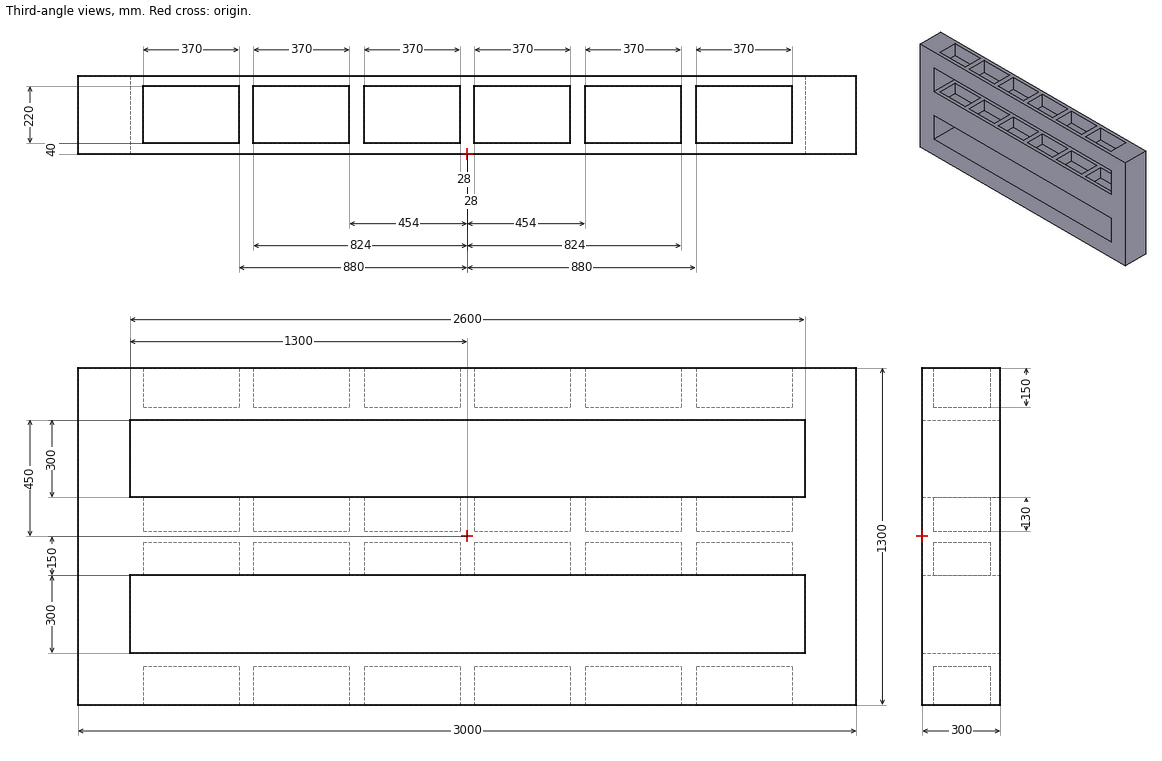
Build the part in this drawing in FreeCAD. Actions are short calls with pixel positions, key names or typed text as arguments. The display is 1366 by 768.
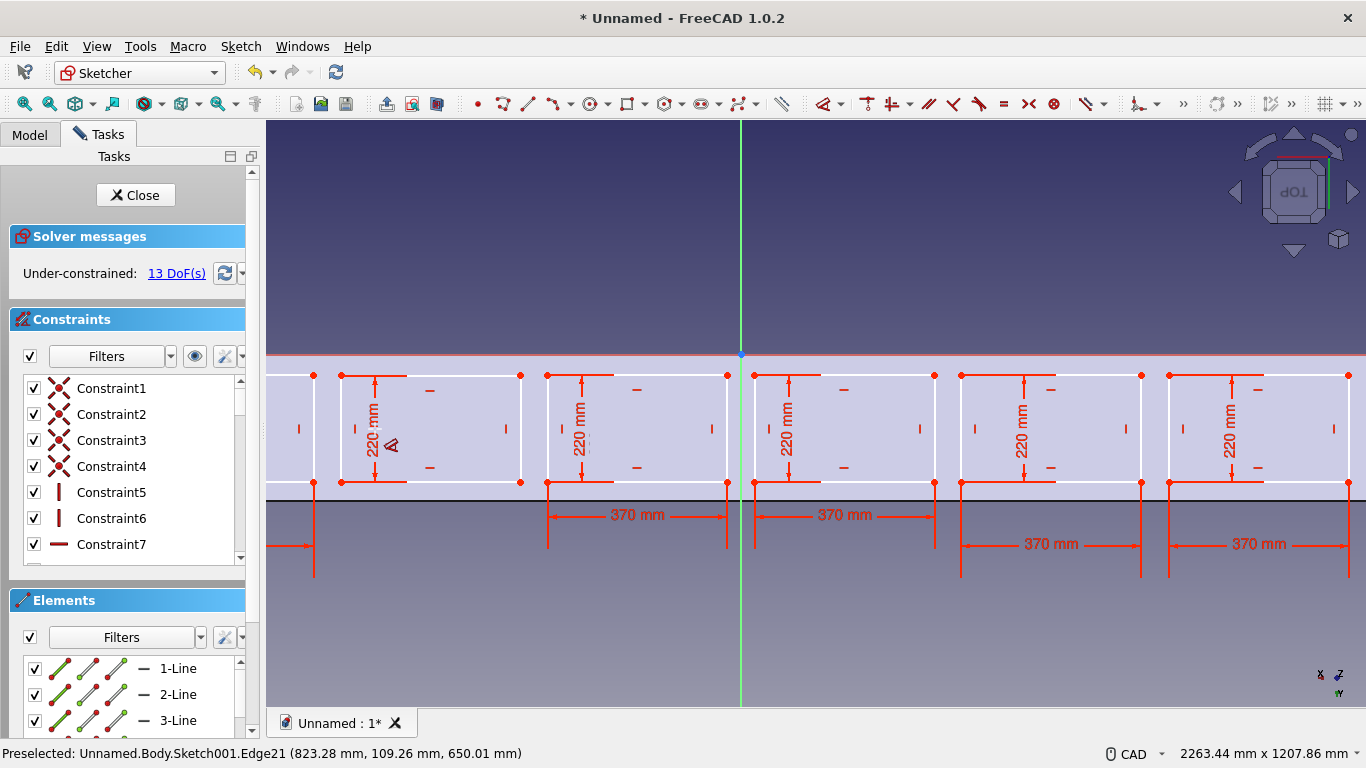
click(395, 482)
click(431, 516)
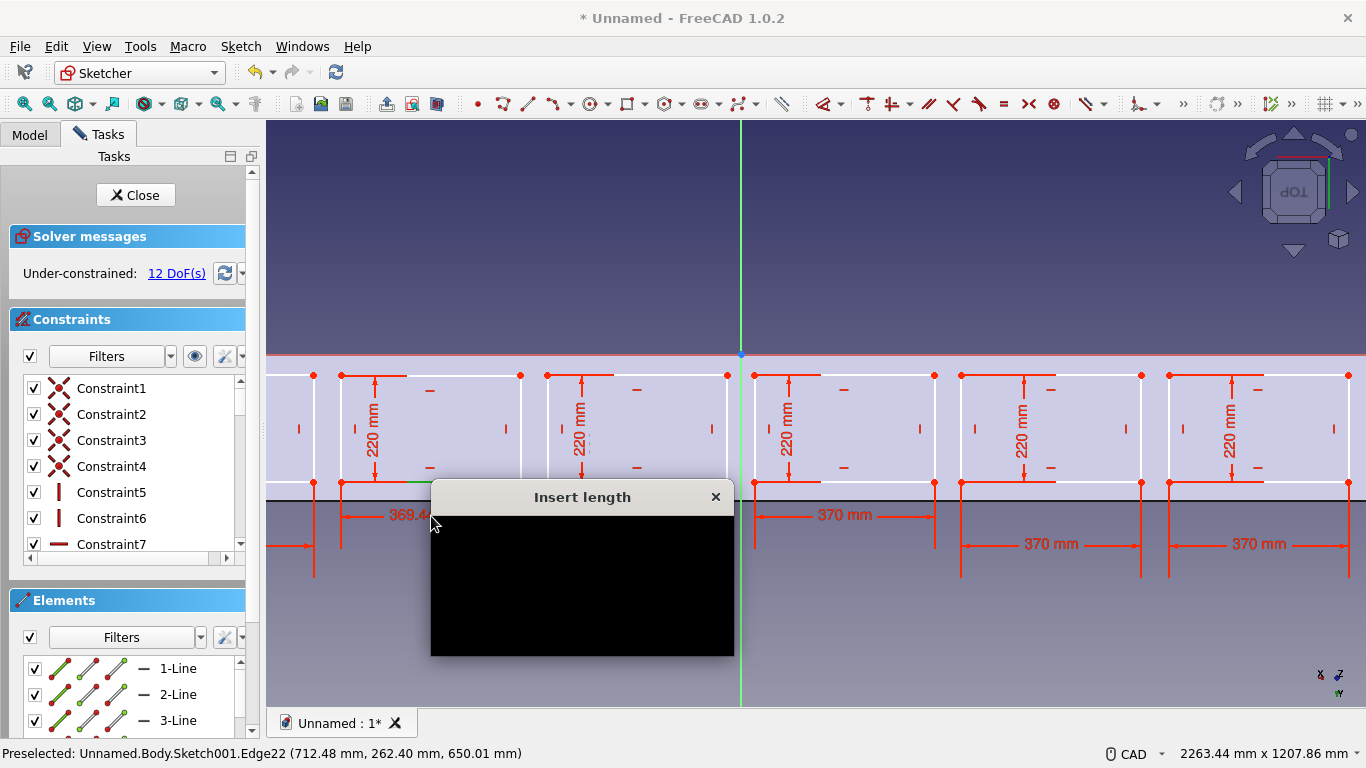
text(370)
key(Return)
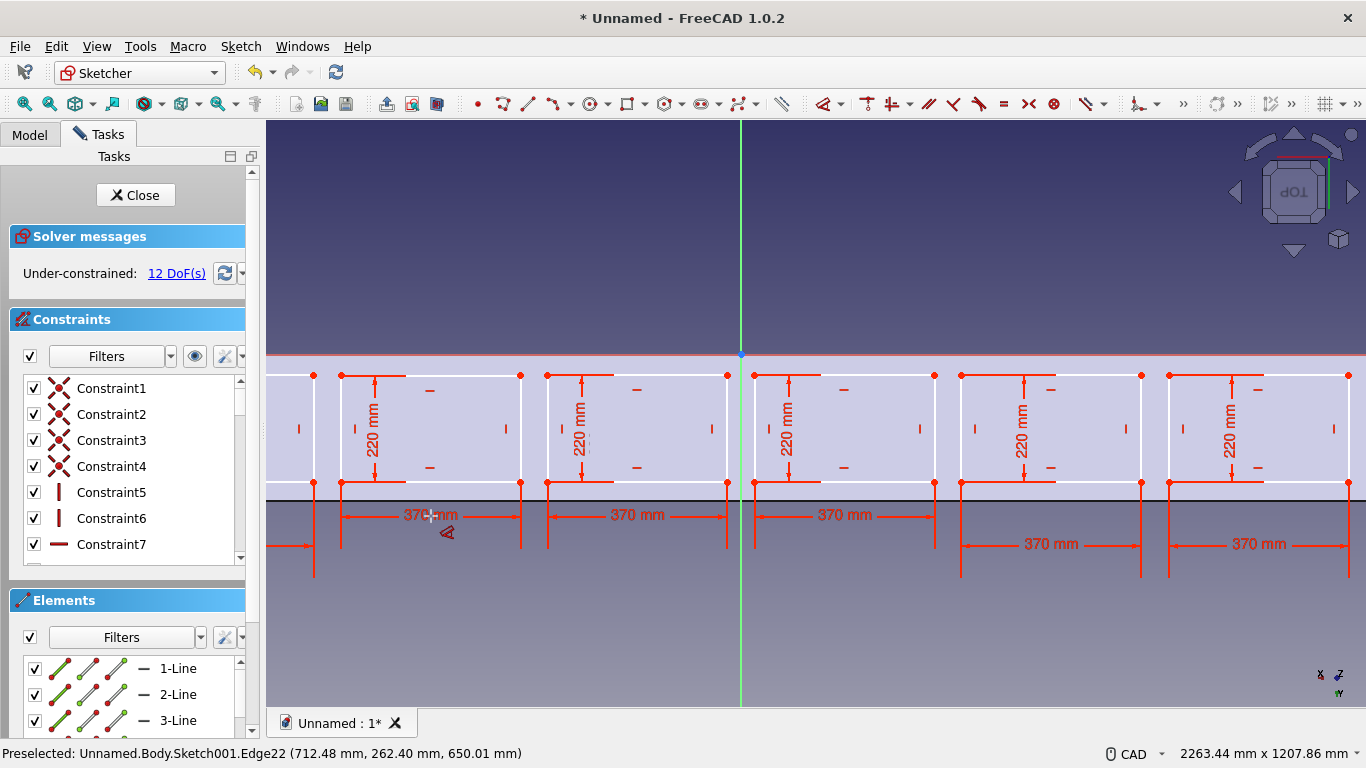
scroll(1169, 375, up, 4)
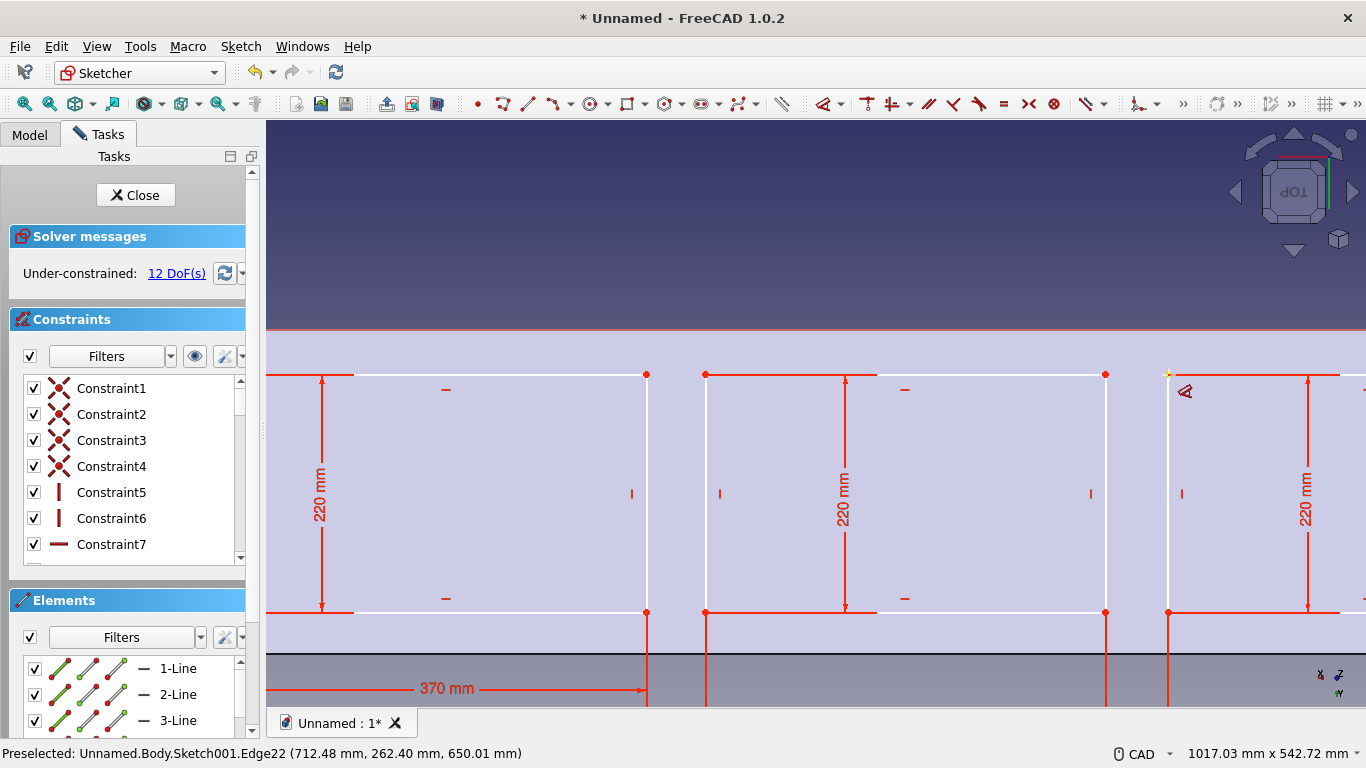
click(1168, 375)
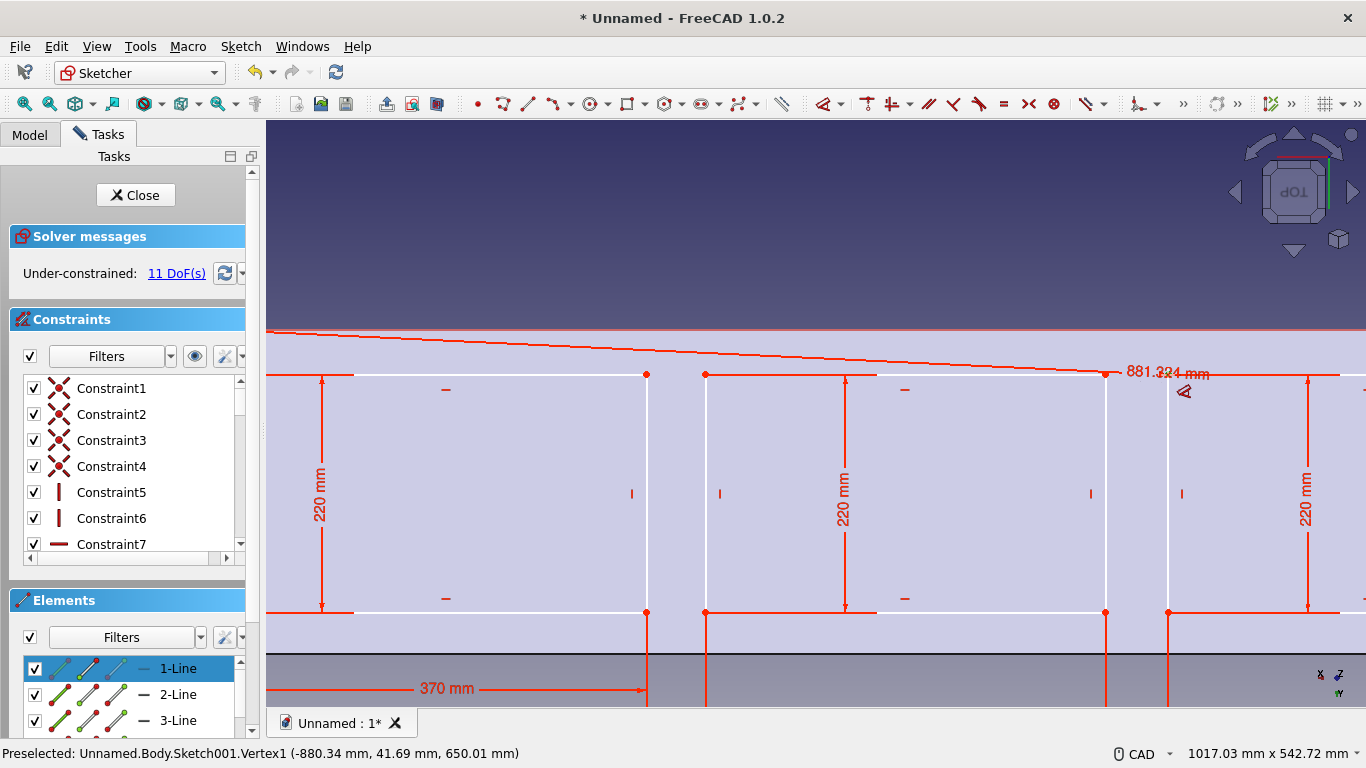
key(Escape)
key(Escape)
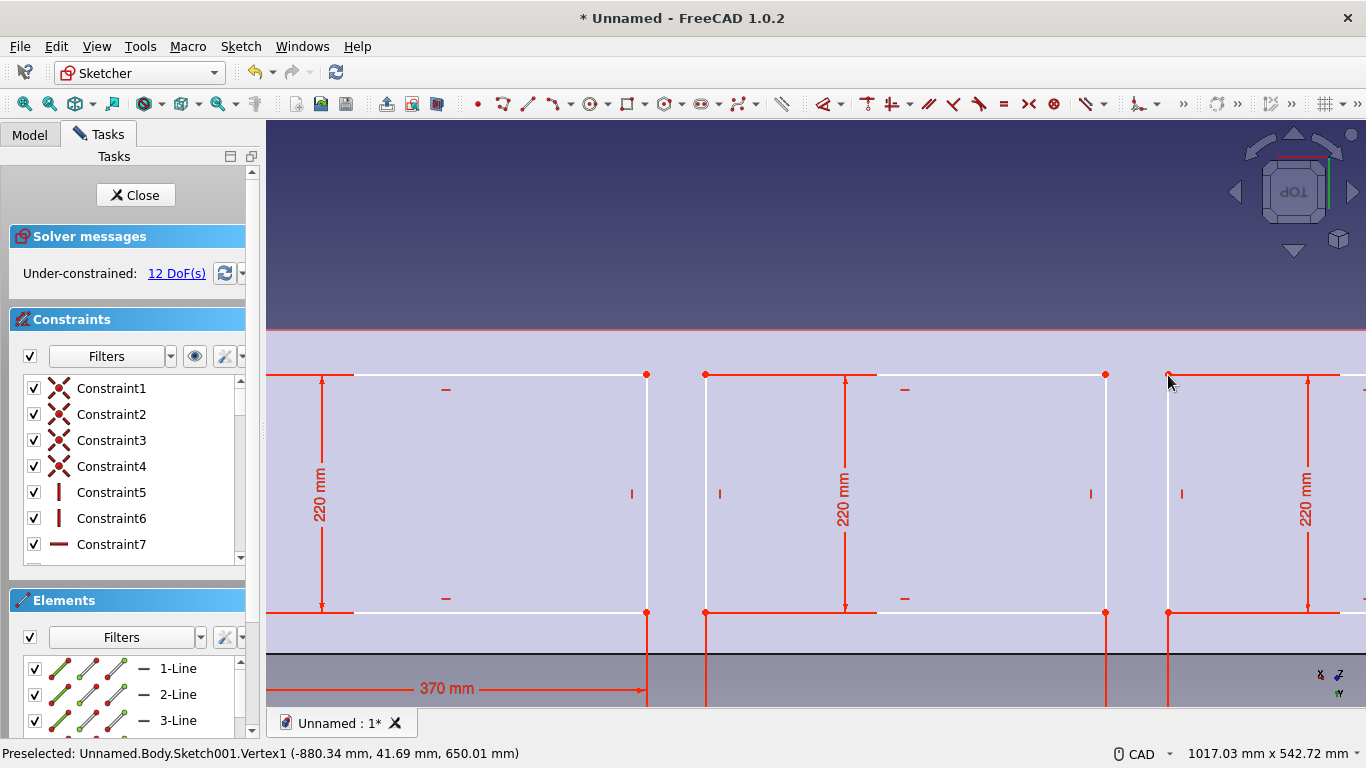
click(1168, 375)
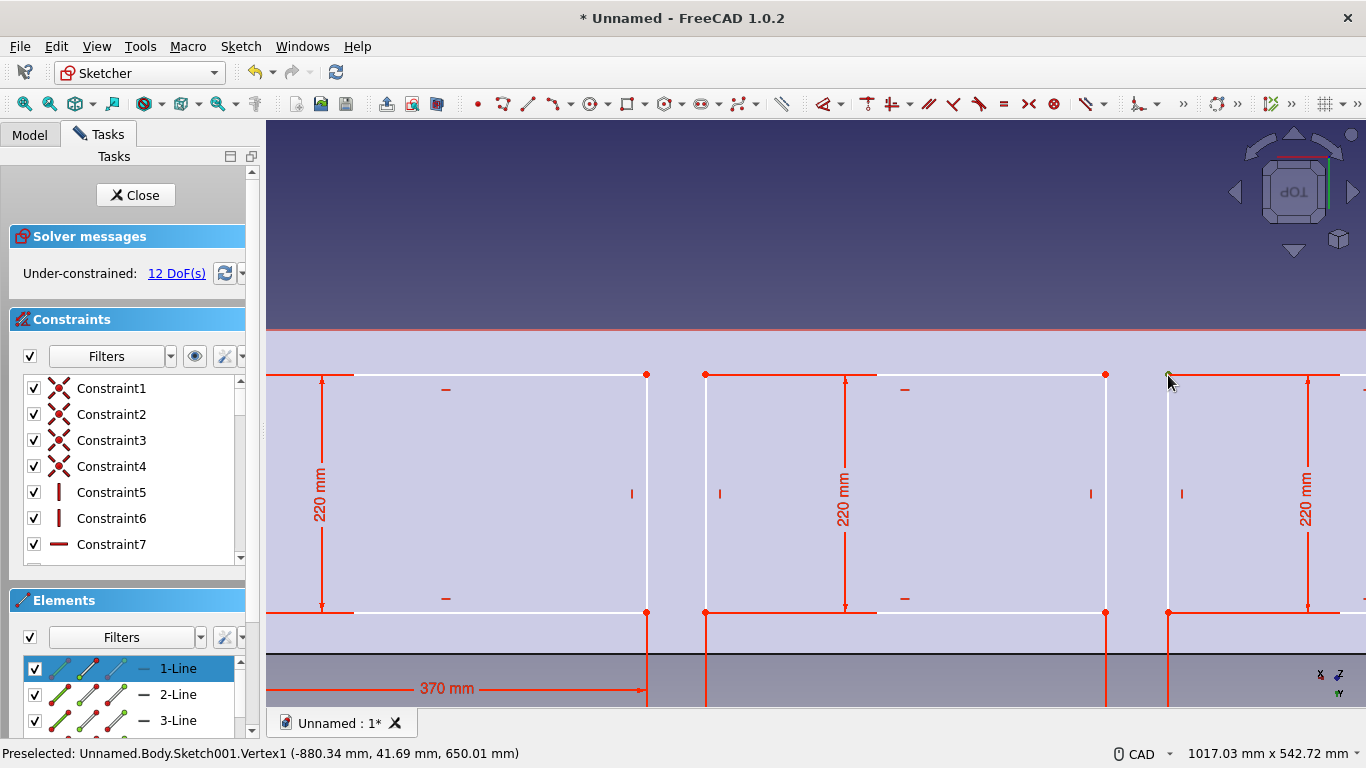
click(840, 104)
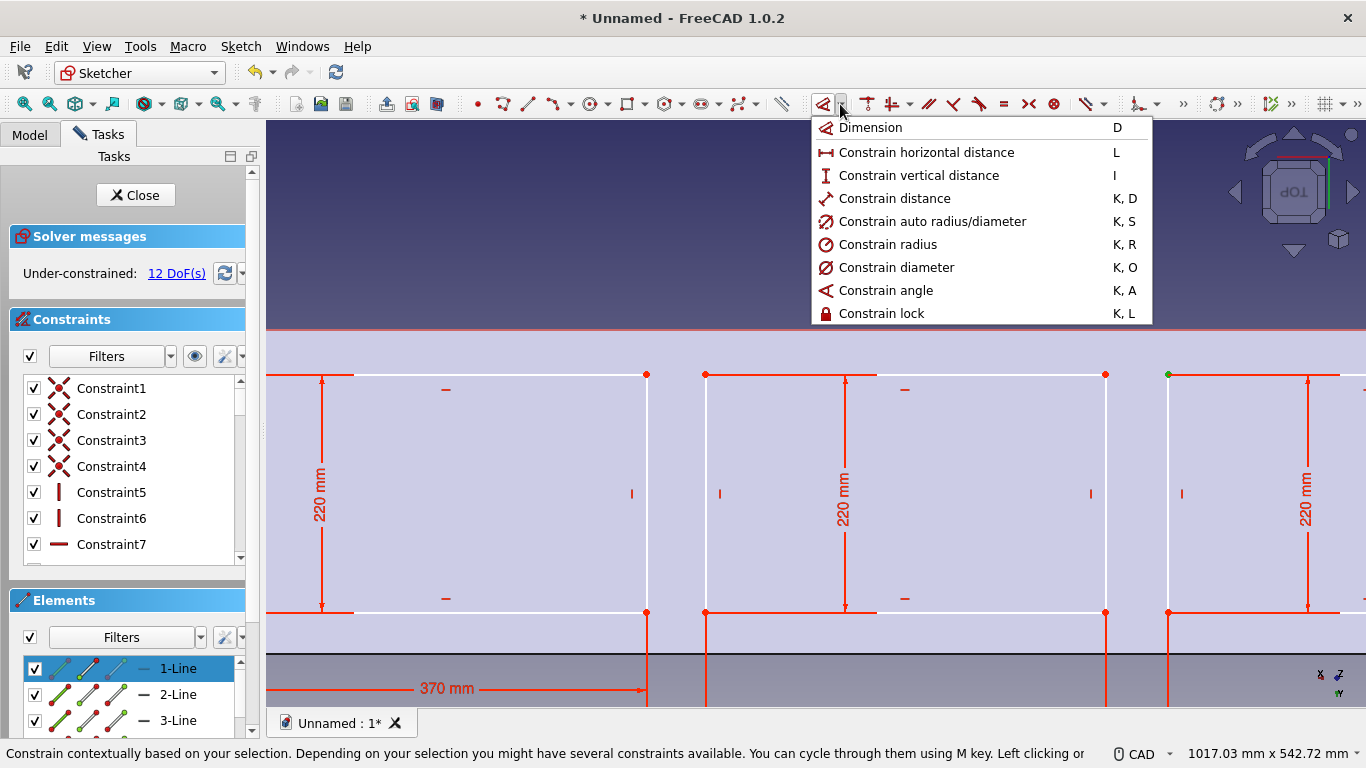
click(982, 176)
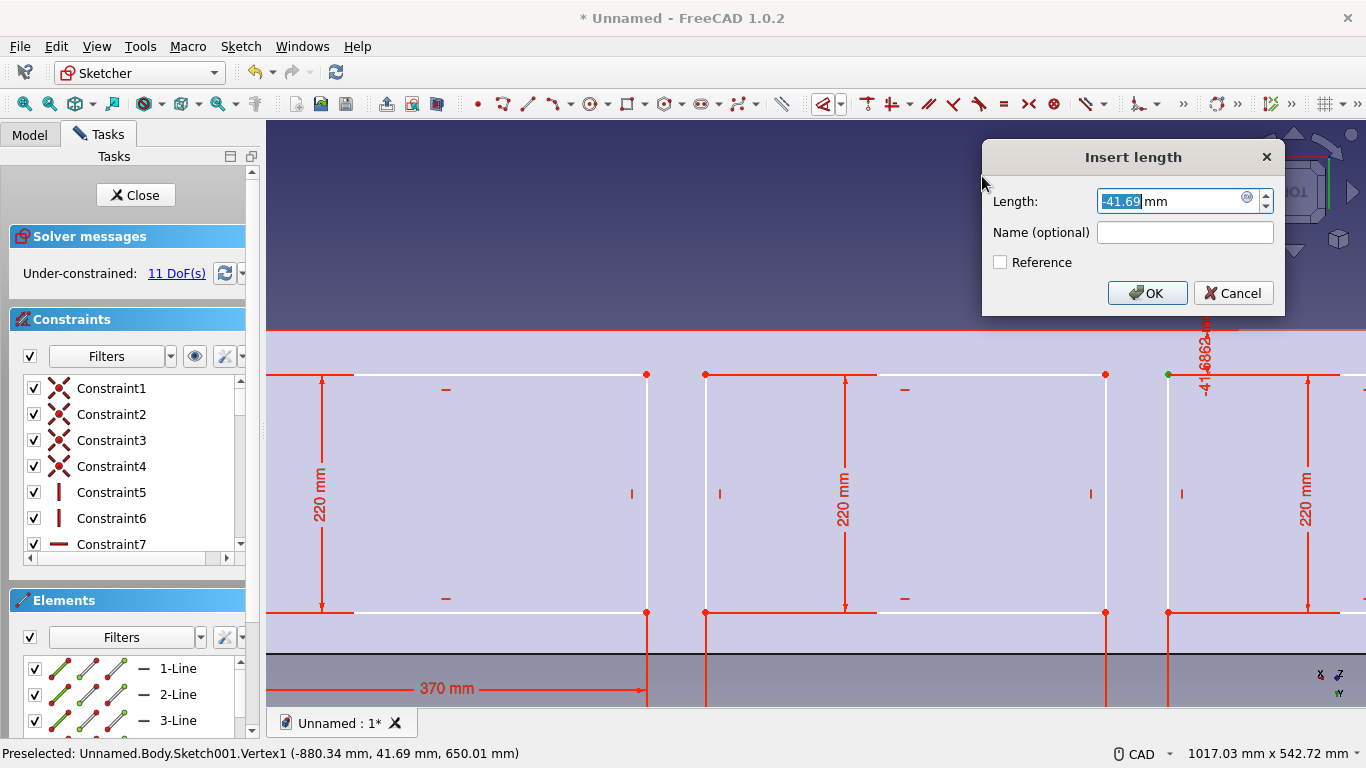
text(-40)
key(Return)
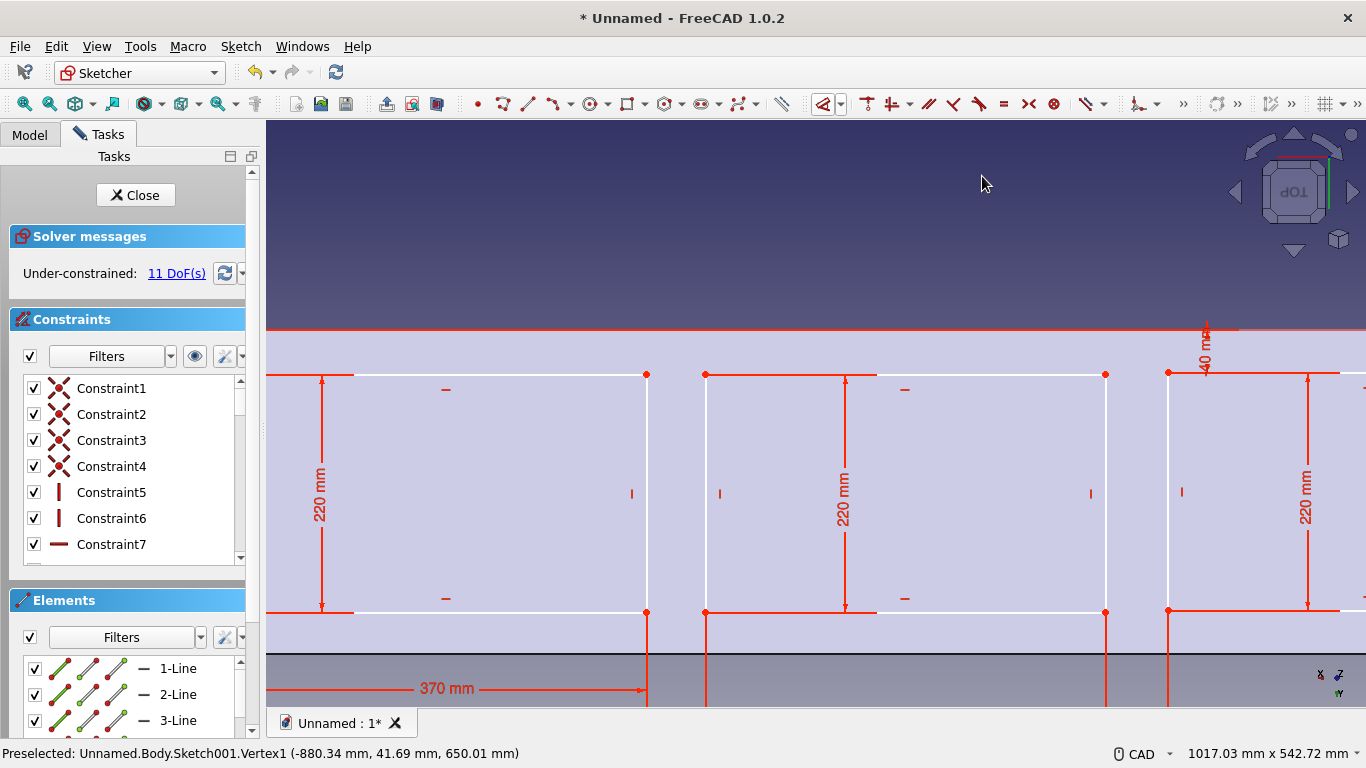
scroll(921, 395, down, 7)